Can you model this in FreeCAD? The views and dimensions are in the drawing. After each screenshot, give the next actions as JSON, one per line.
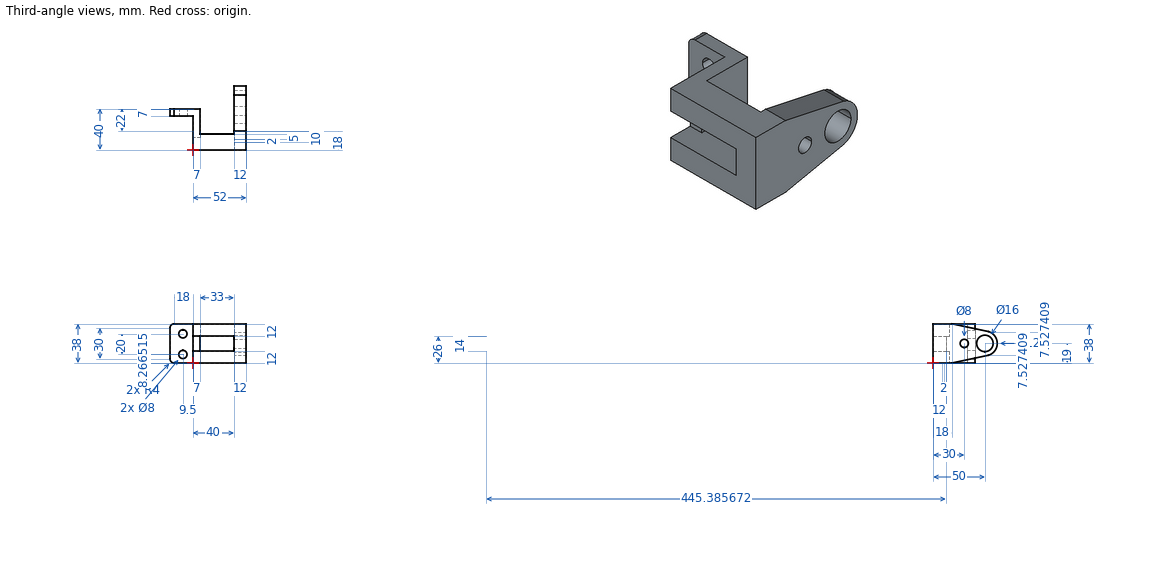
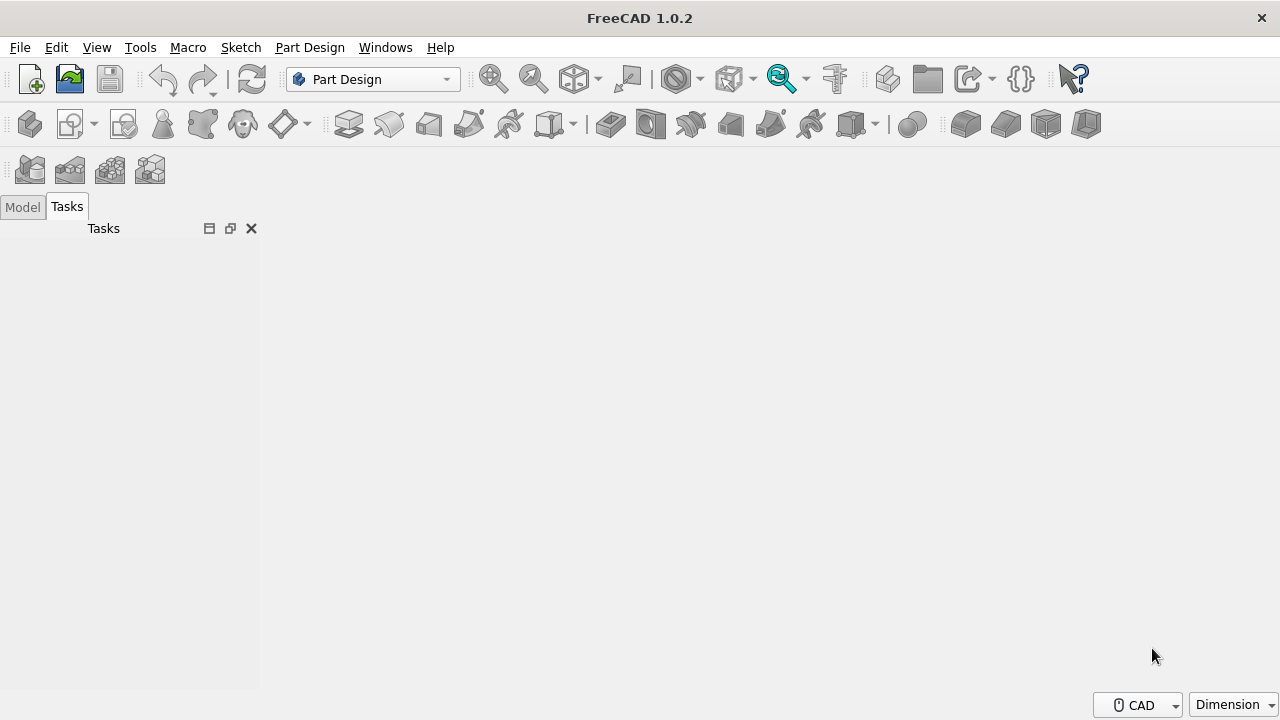
{"action": "left_click", "coordinate": [30, 80]}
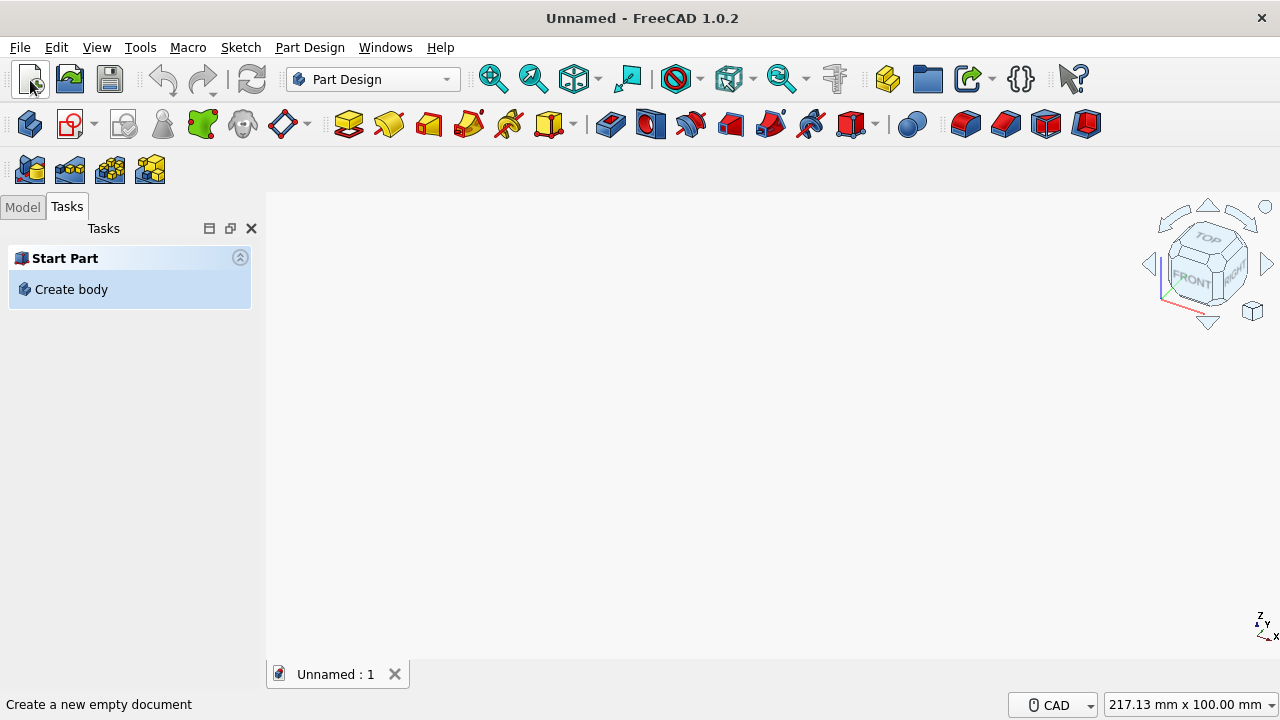
{"action": "left_click", "coordinate": [70, 124]}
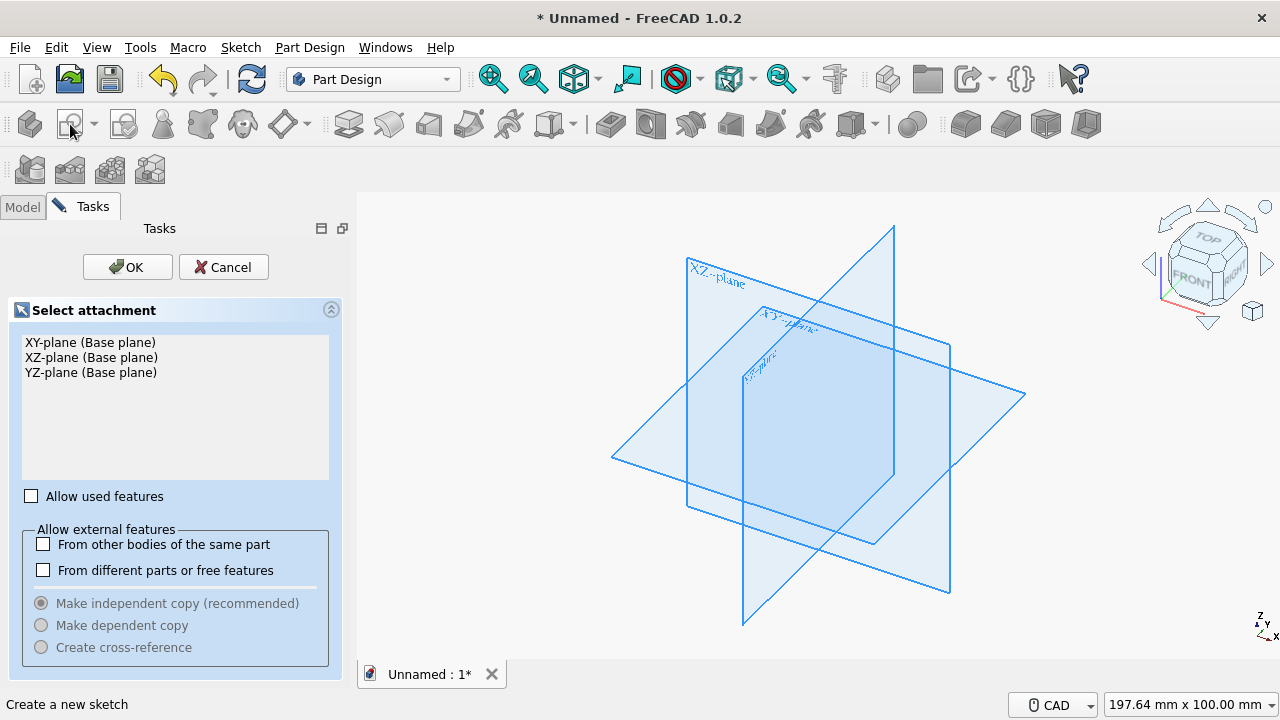
{"action": "left_click", "coordinate": [82, 342]}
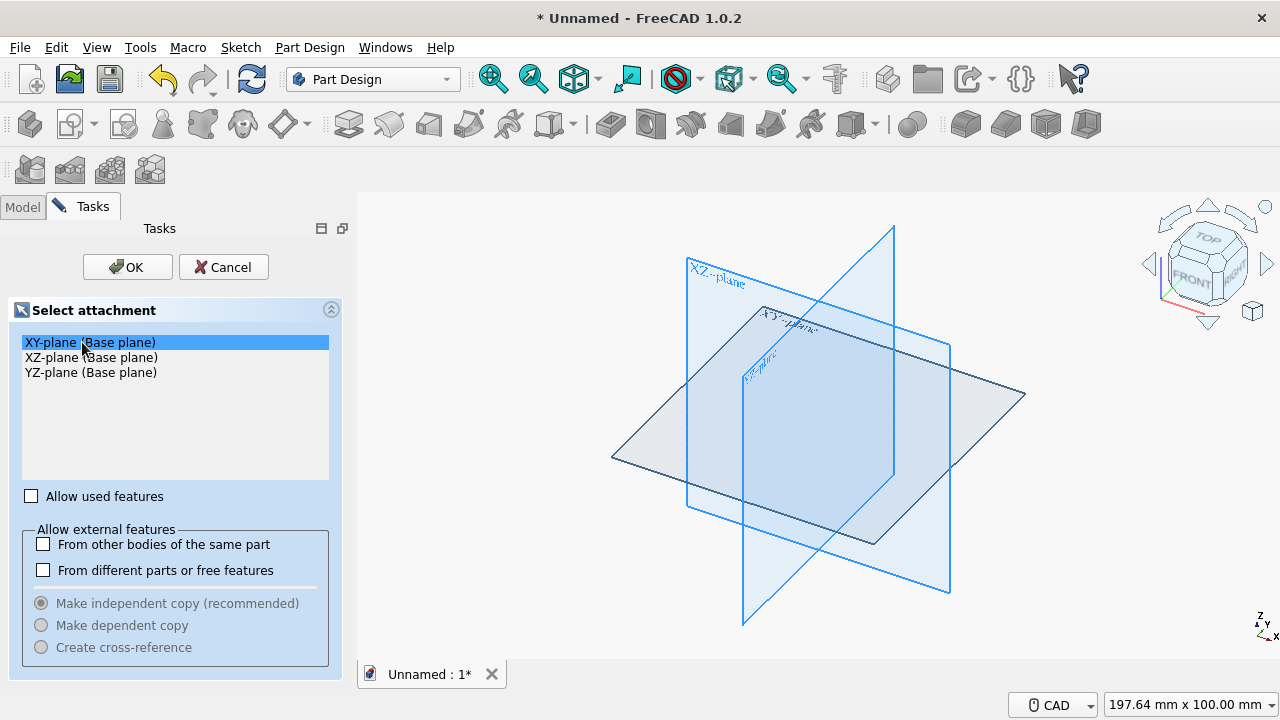
{"action": "left_click", "coordinate": [128, 267]}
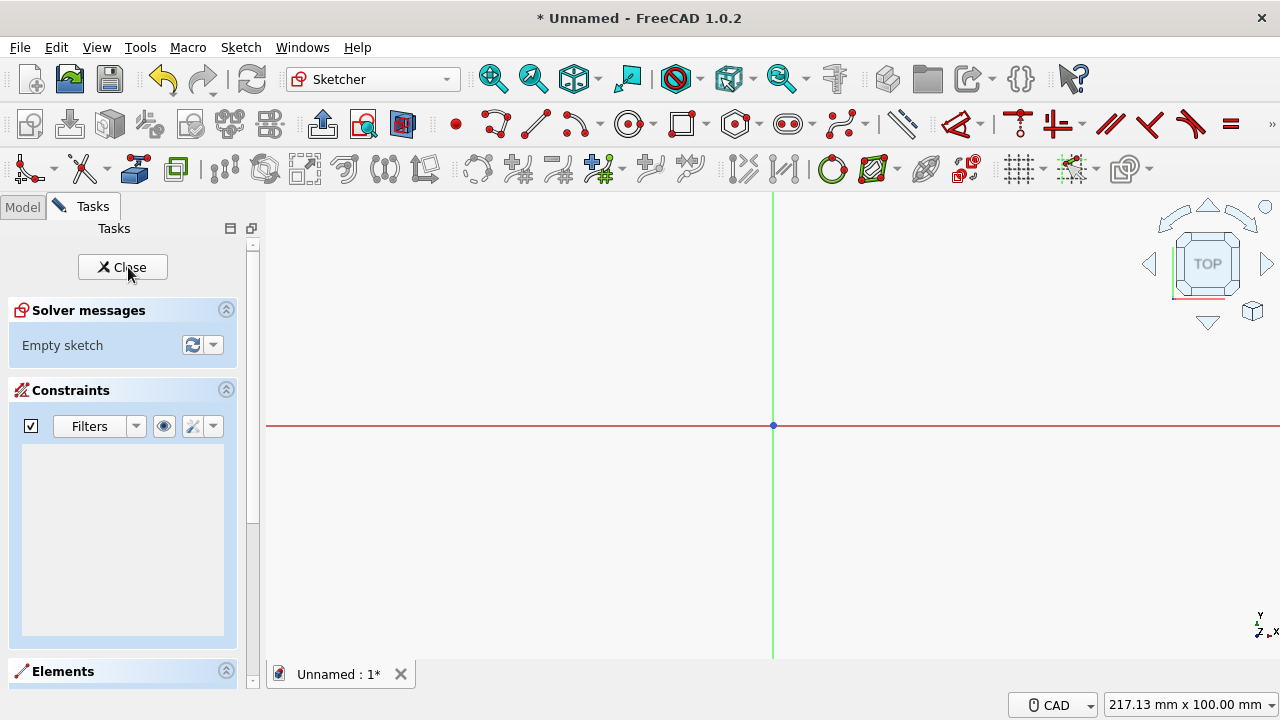
{"action": "scroll", "coordinate": [1049, 349], "scroll_direction": "up", "scroll_amount": 4}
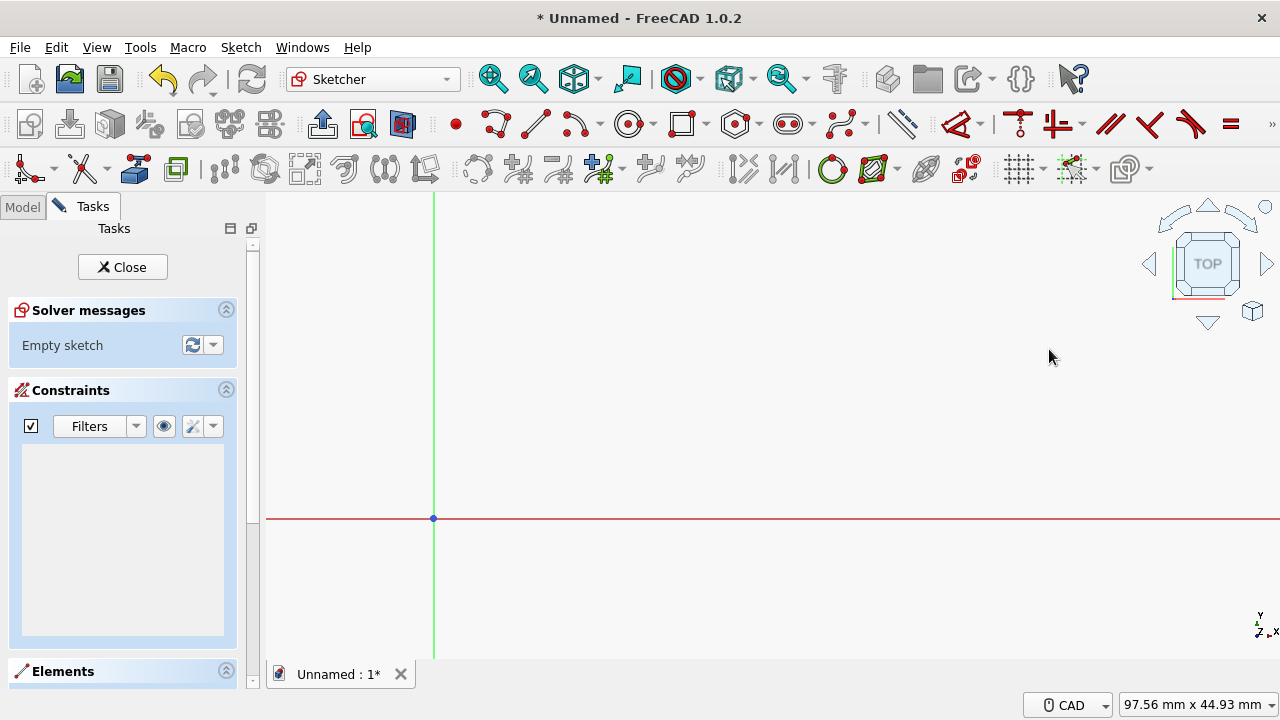
{"action": "left_click", "coordinate": [496, 124]}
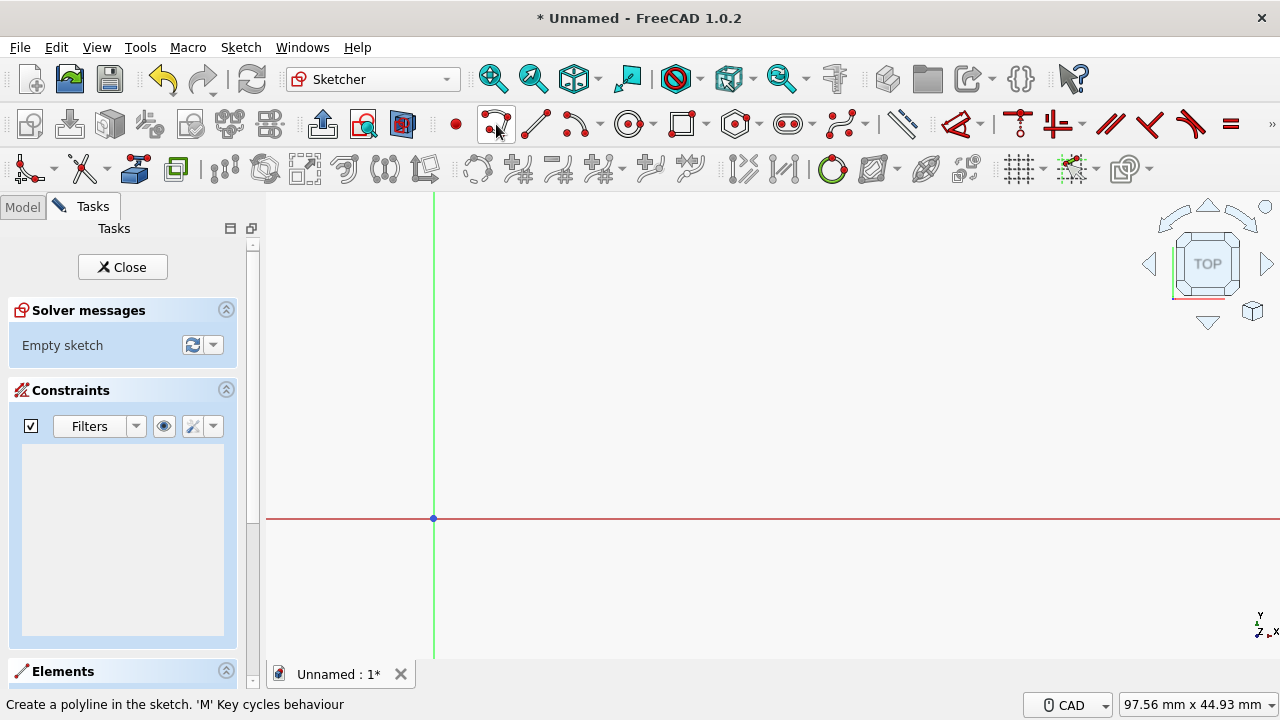
{"action": "left_click", "coordinate": [434, 519]}
{"action": "left_click", "coordinate": [974, 510]}
{"action": "left_click", "coordinate": [974, 332]}
{"action": "left_click", "coordinate": [850, 332]}
{"action": "left_click", "coordinate": [850, 436]}
{"action": "left_click", "coordinate": [507, 436]}
{"action": "left_click", "coordinate": [507, 332]}
{"action": "left_click", "coordinate": [443, 332]}
{"action": "left_click", "coordinate": [434, 519]}
{"action": "key", "text": "Escape"}
{"action": "key", "text": "Escape"}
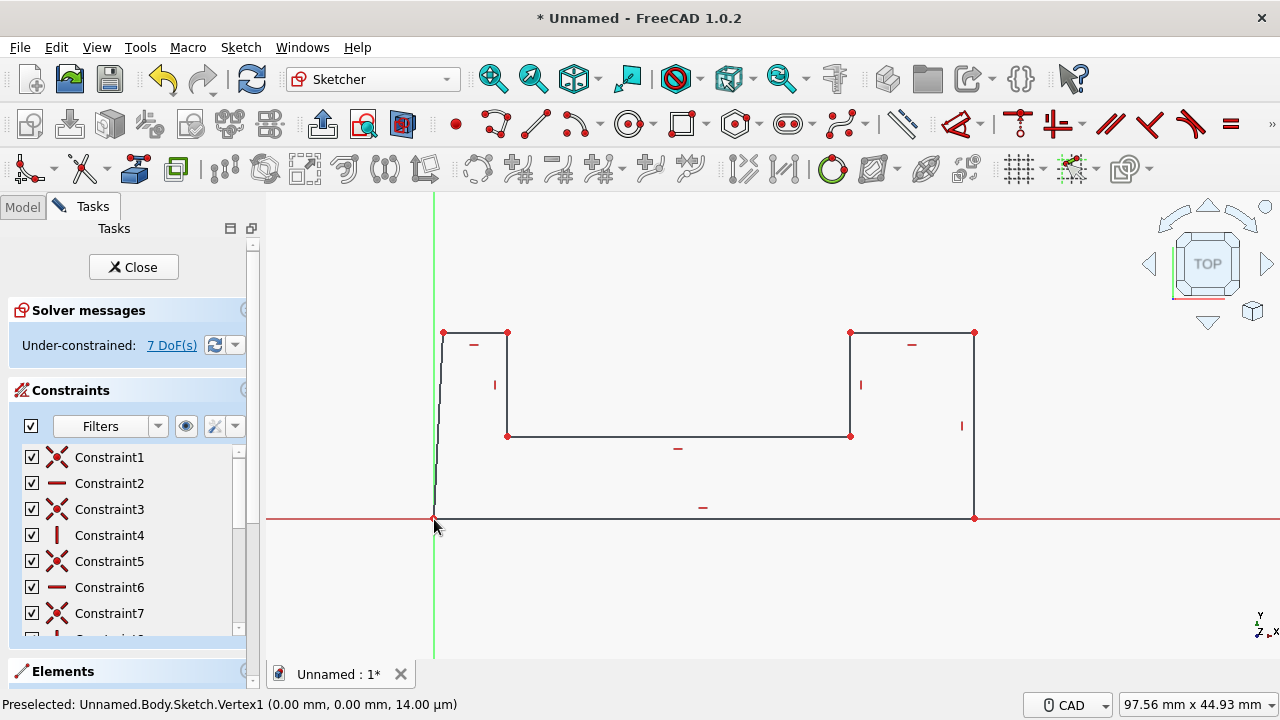
{"action": "left_click", "coordinate": [437, 463]}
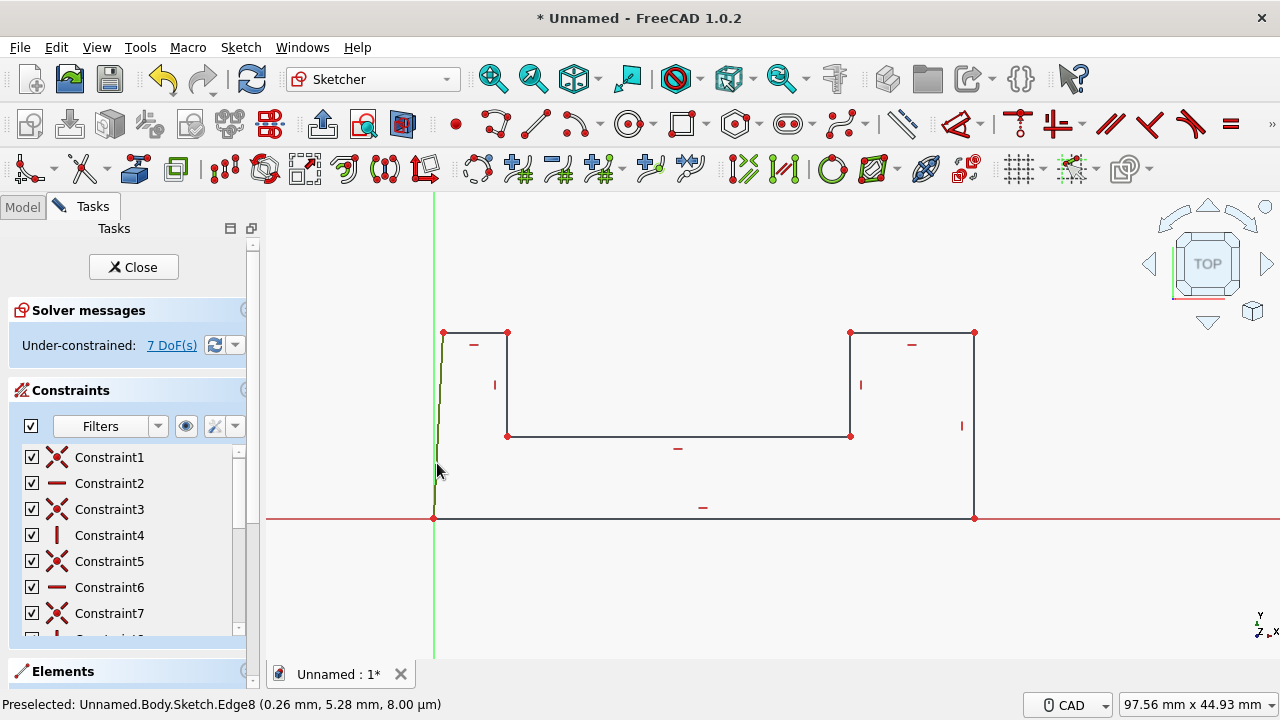
{"action": "left_click", "coordinate": [1084, 124]}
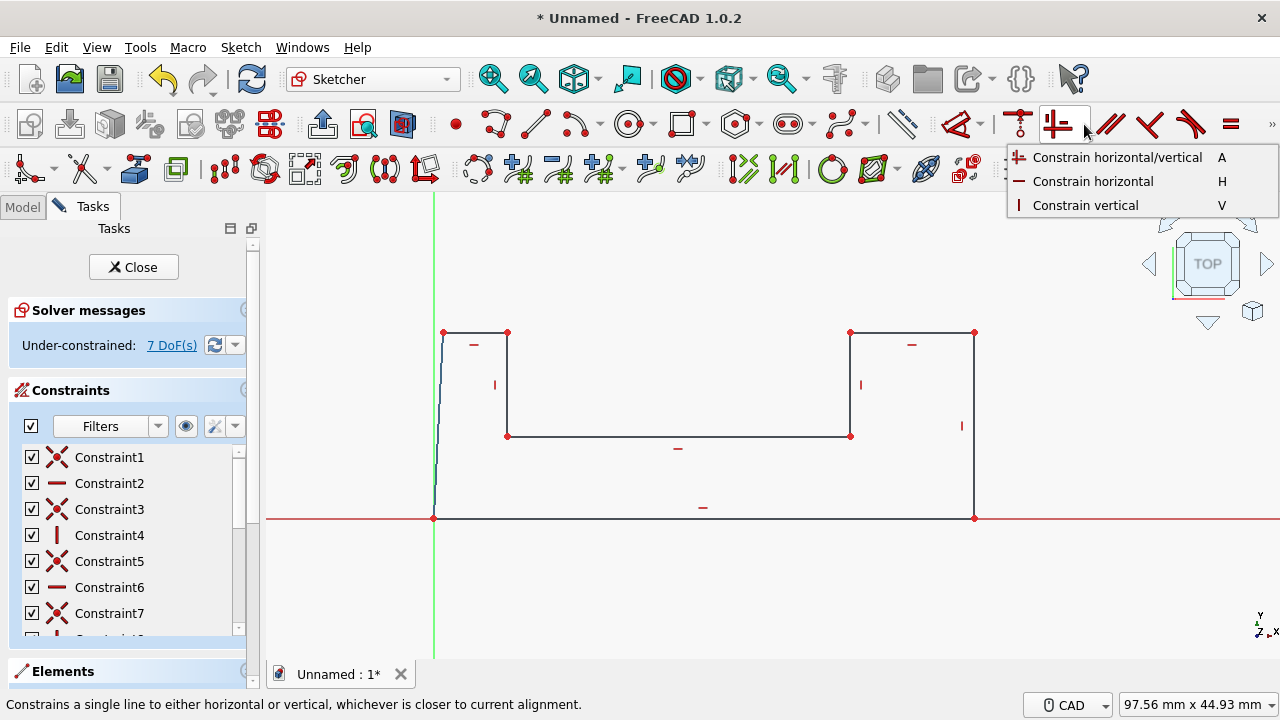
{"action": "left_click", "coordinate": [1143, 205]}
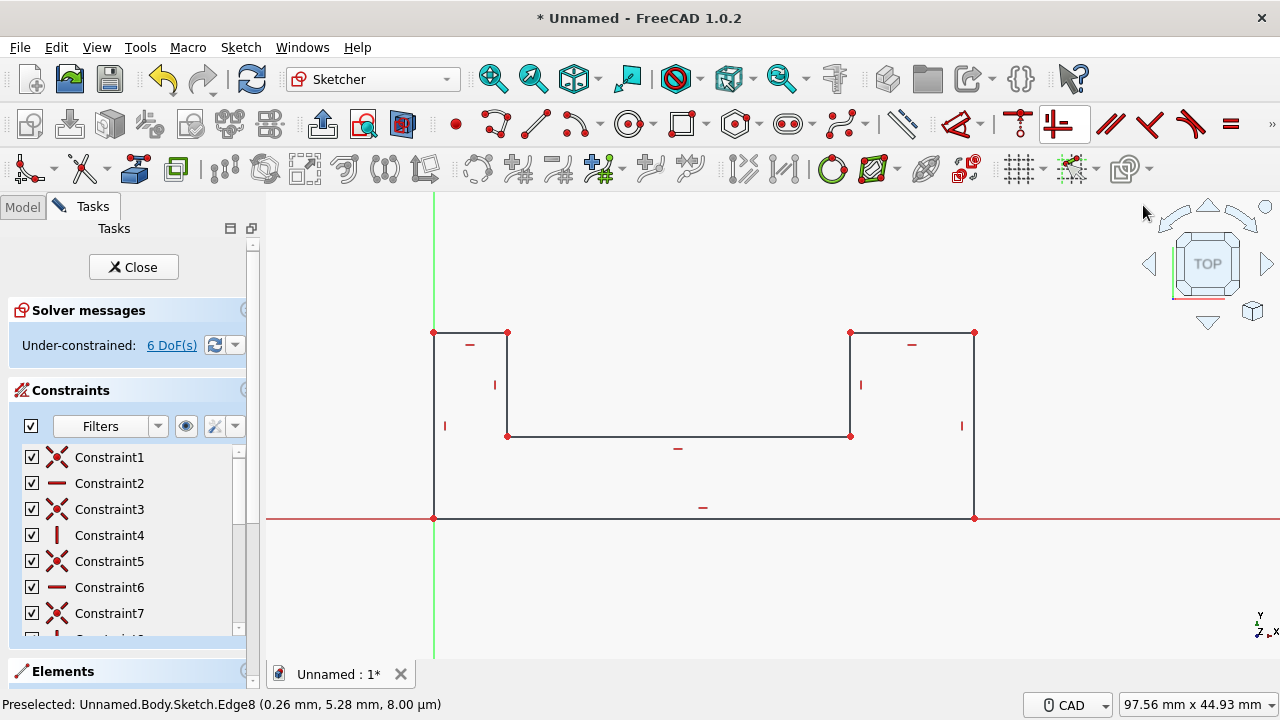
{"action": "left_click", "coordinate": [956, 124]}